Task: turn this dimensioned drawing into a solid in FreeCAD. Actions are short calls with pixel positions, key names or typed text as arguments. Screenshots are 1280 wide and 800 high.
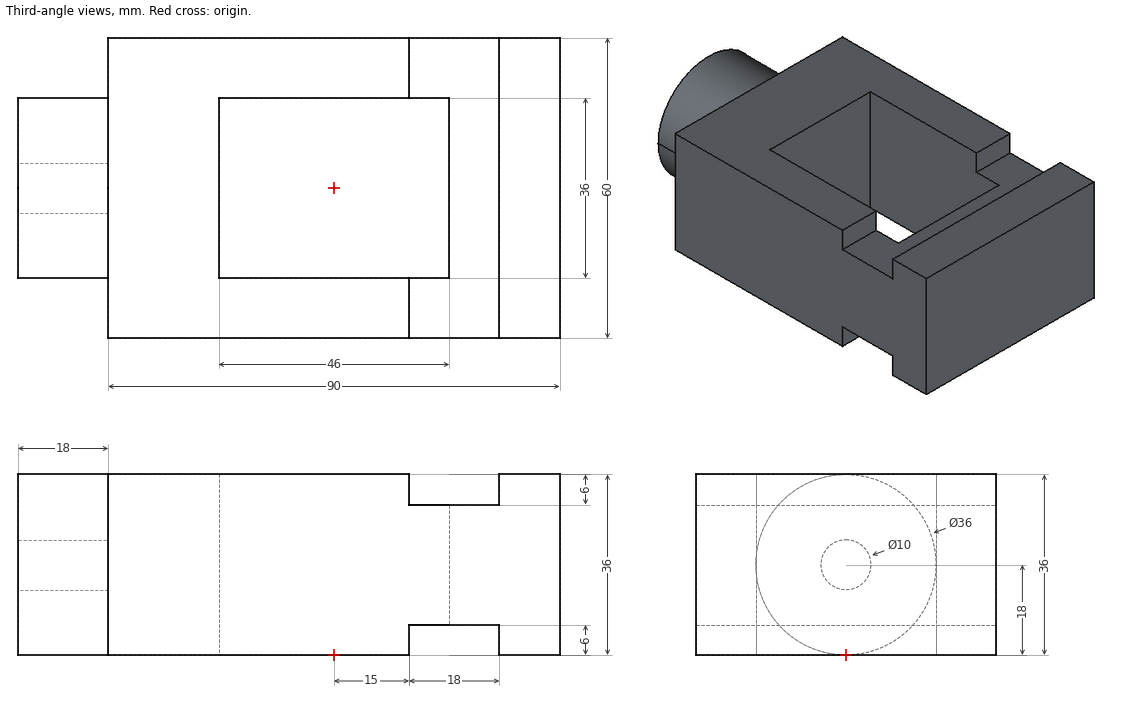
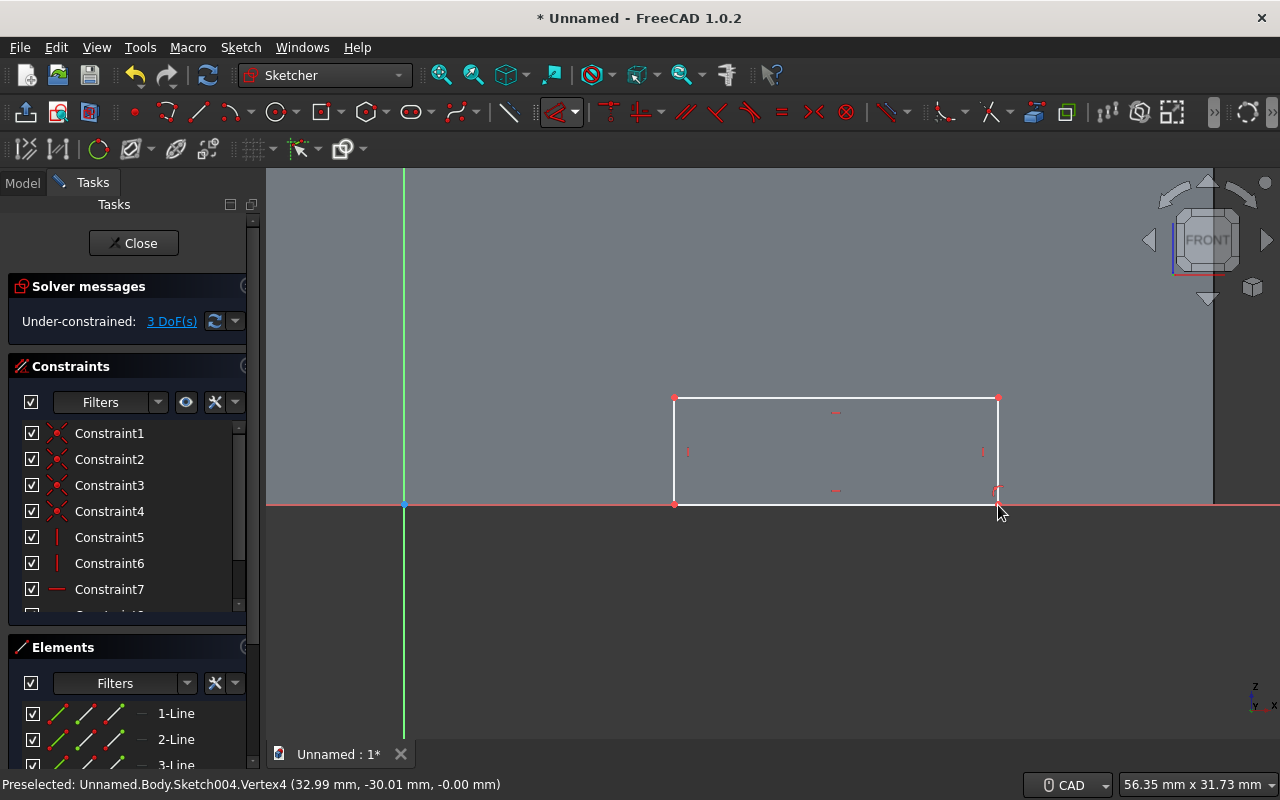
click(674, 430)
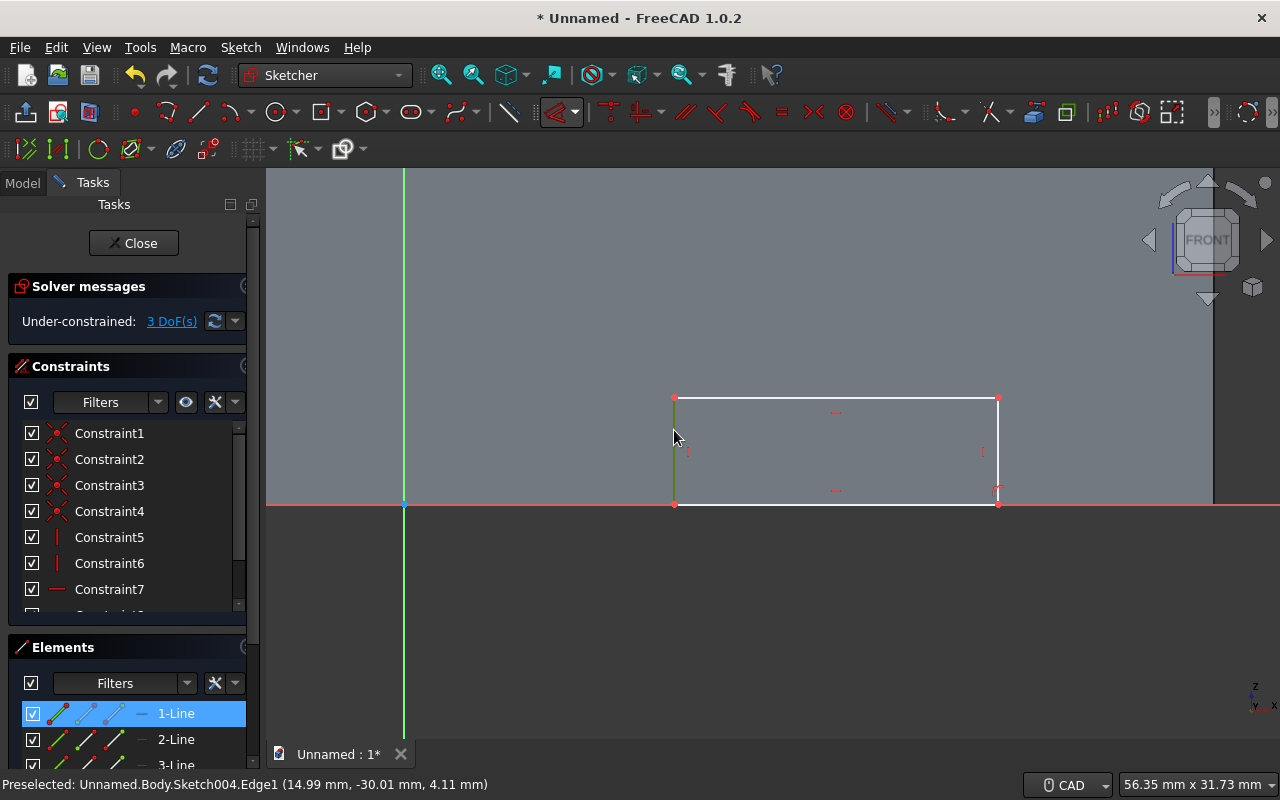
key(i)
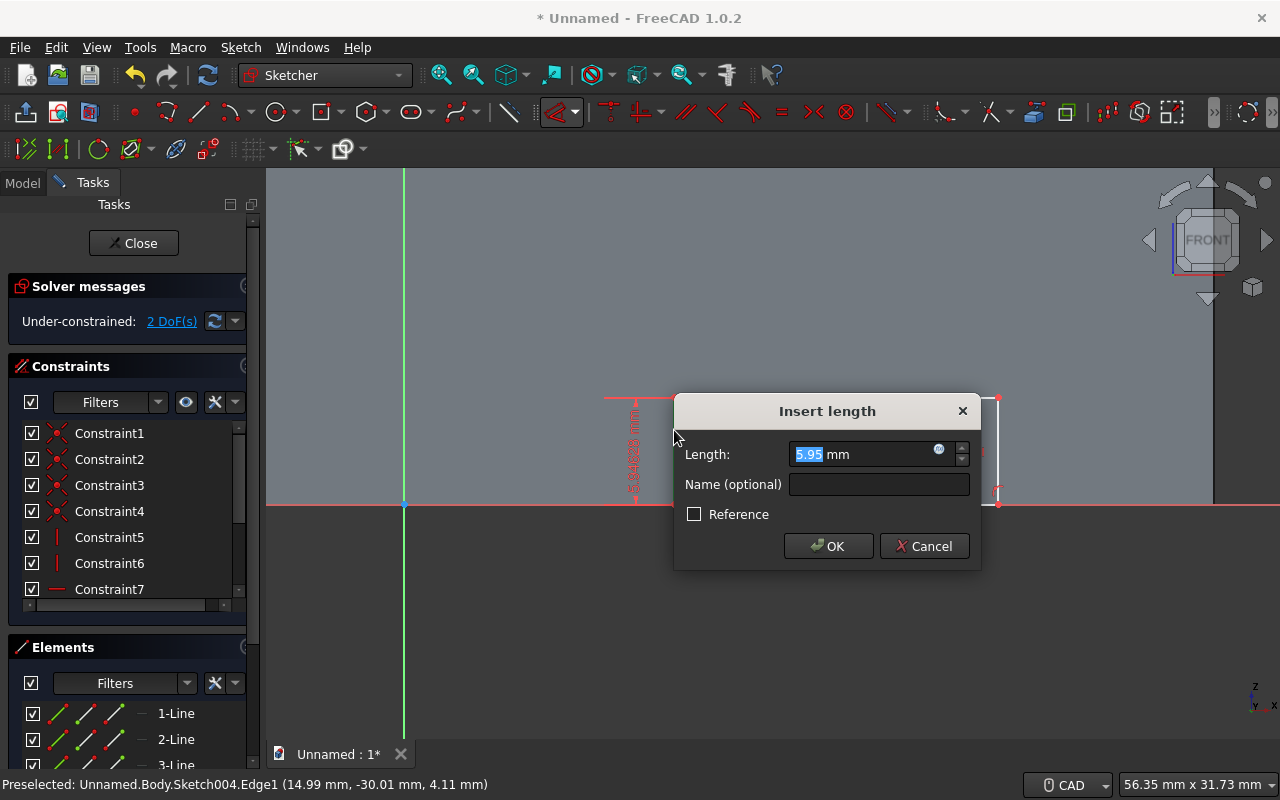
text(6)
key(Return)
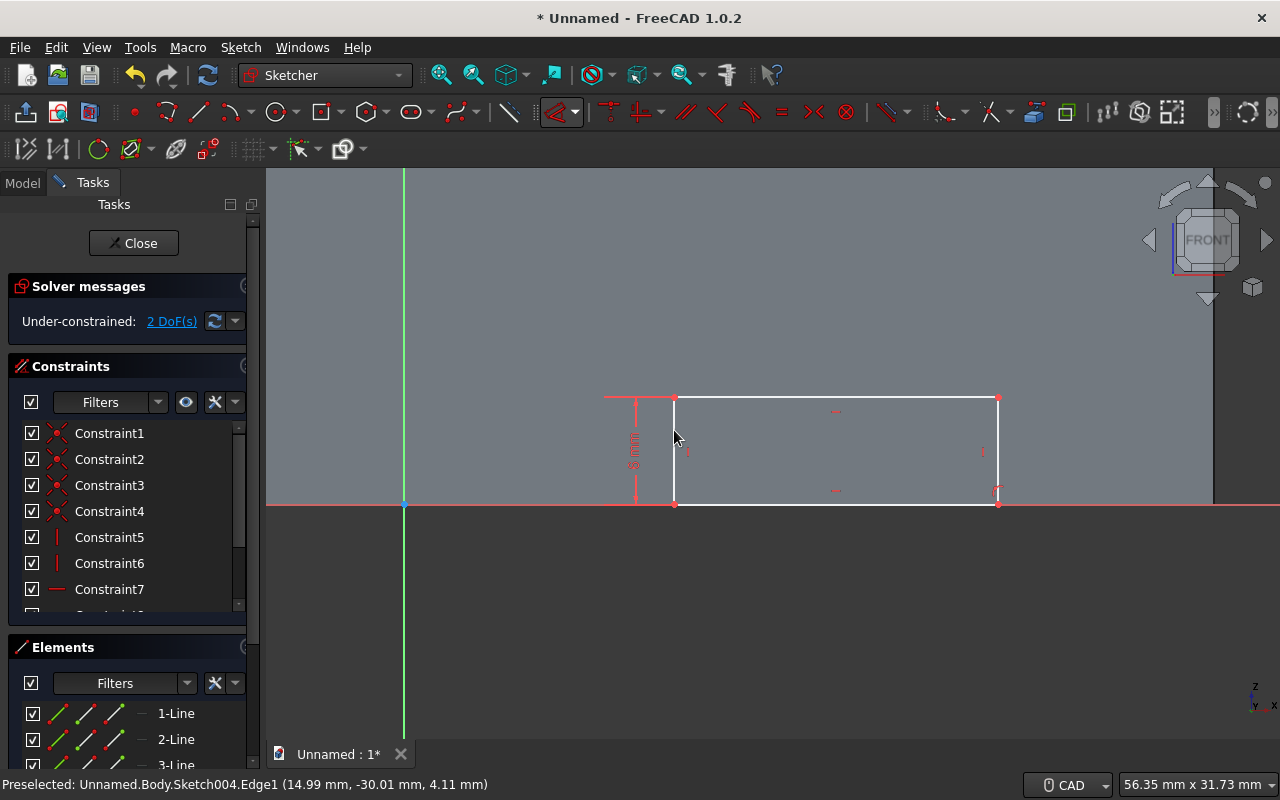
click(771, 505)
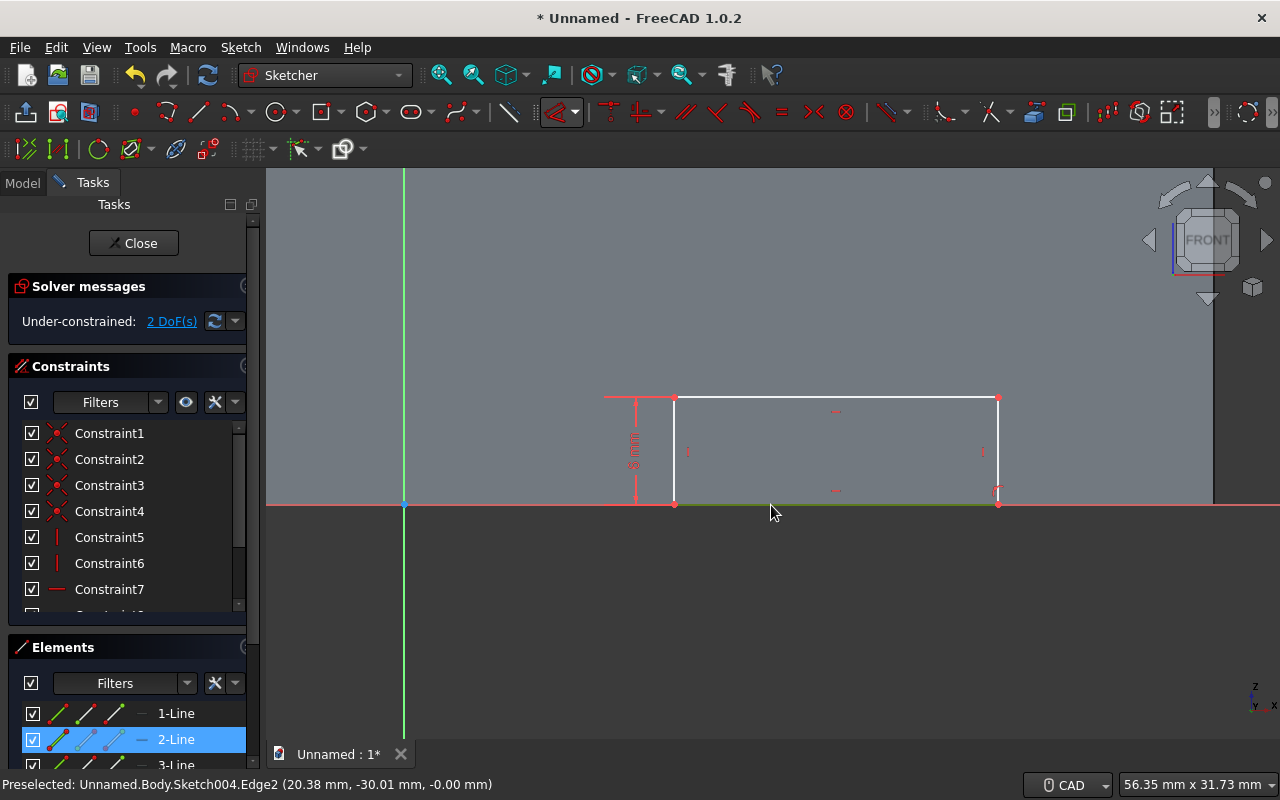
key(l)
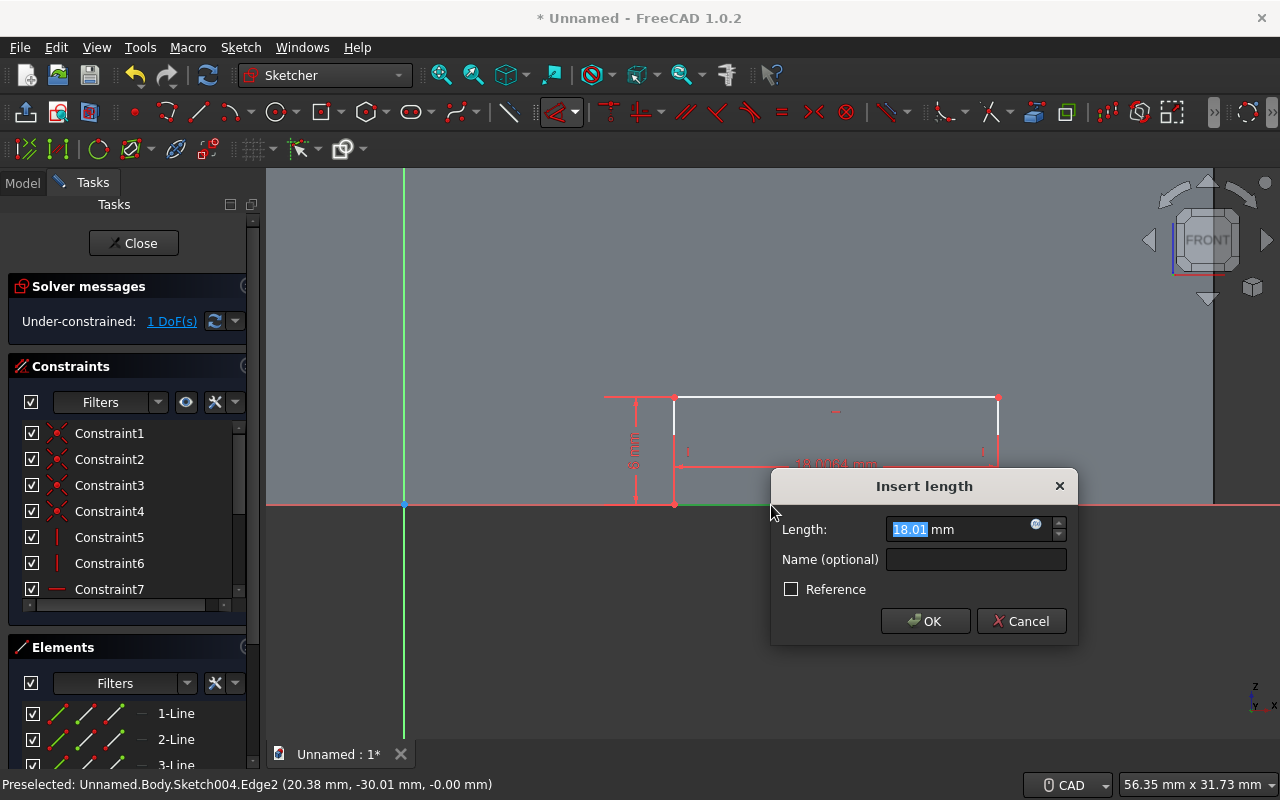
text(18)
key(Return)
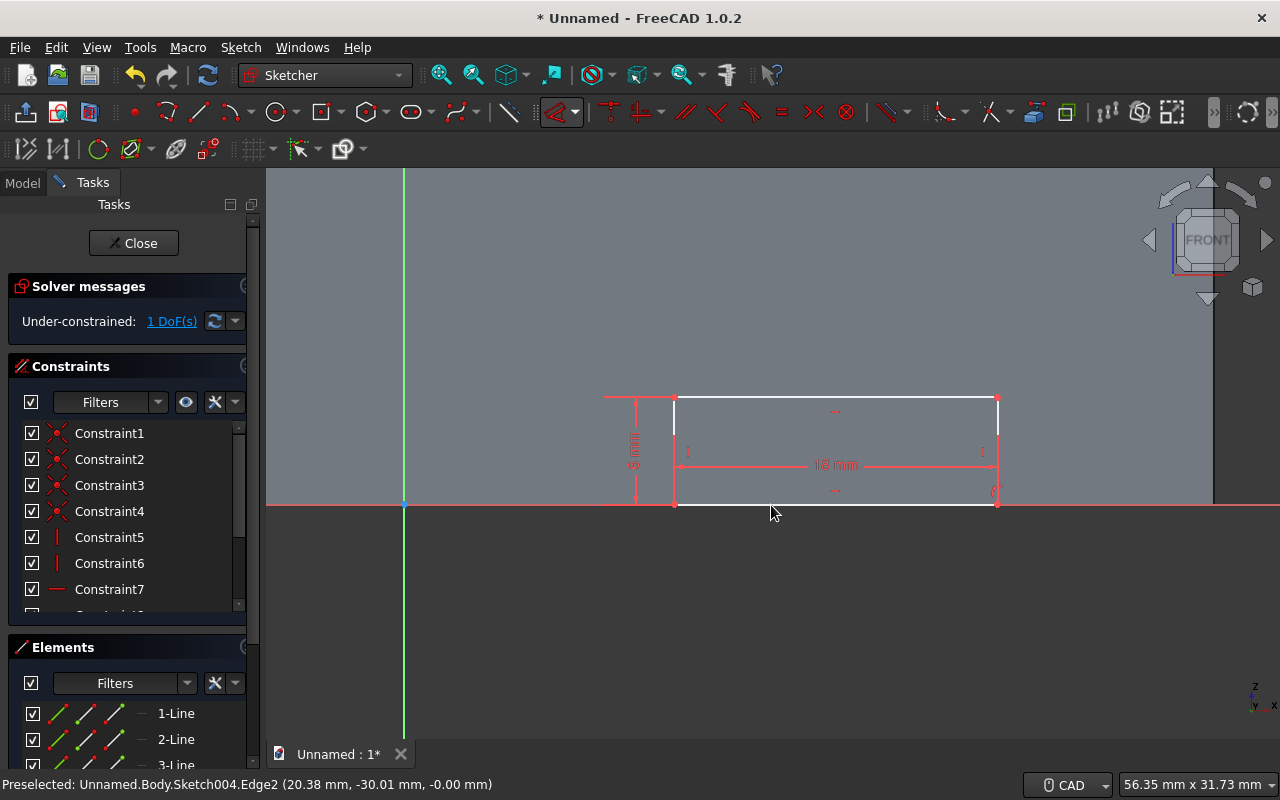
click(674, 397)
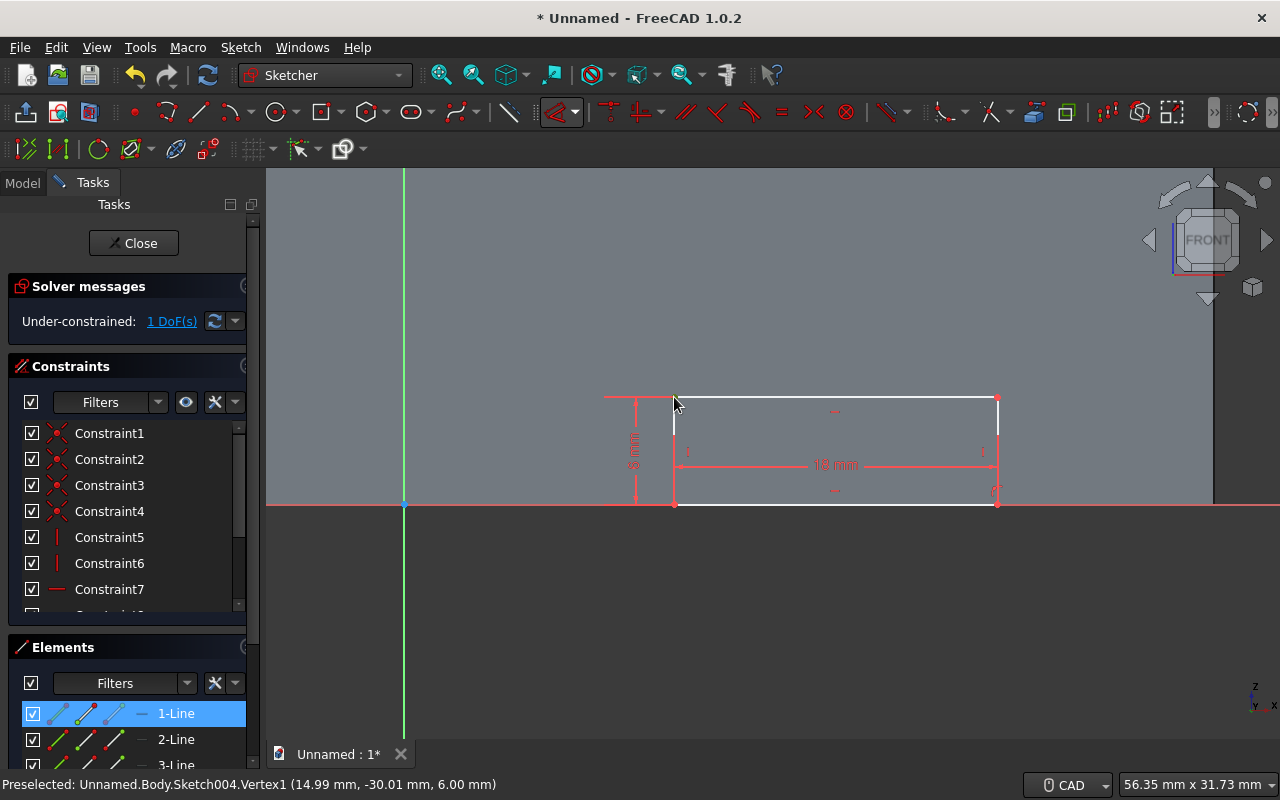
key(l)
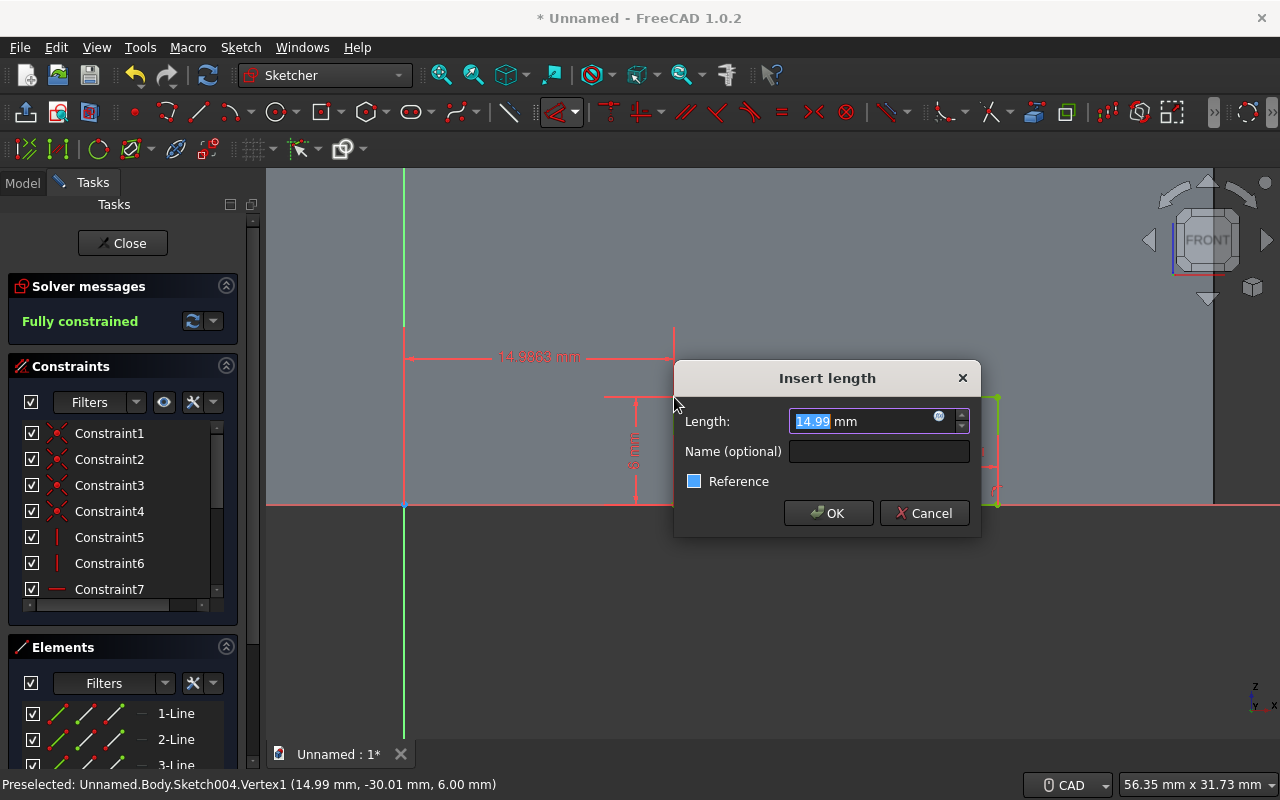
text(15)
key(Return)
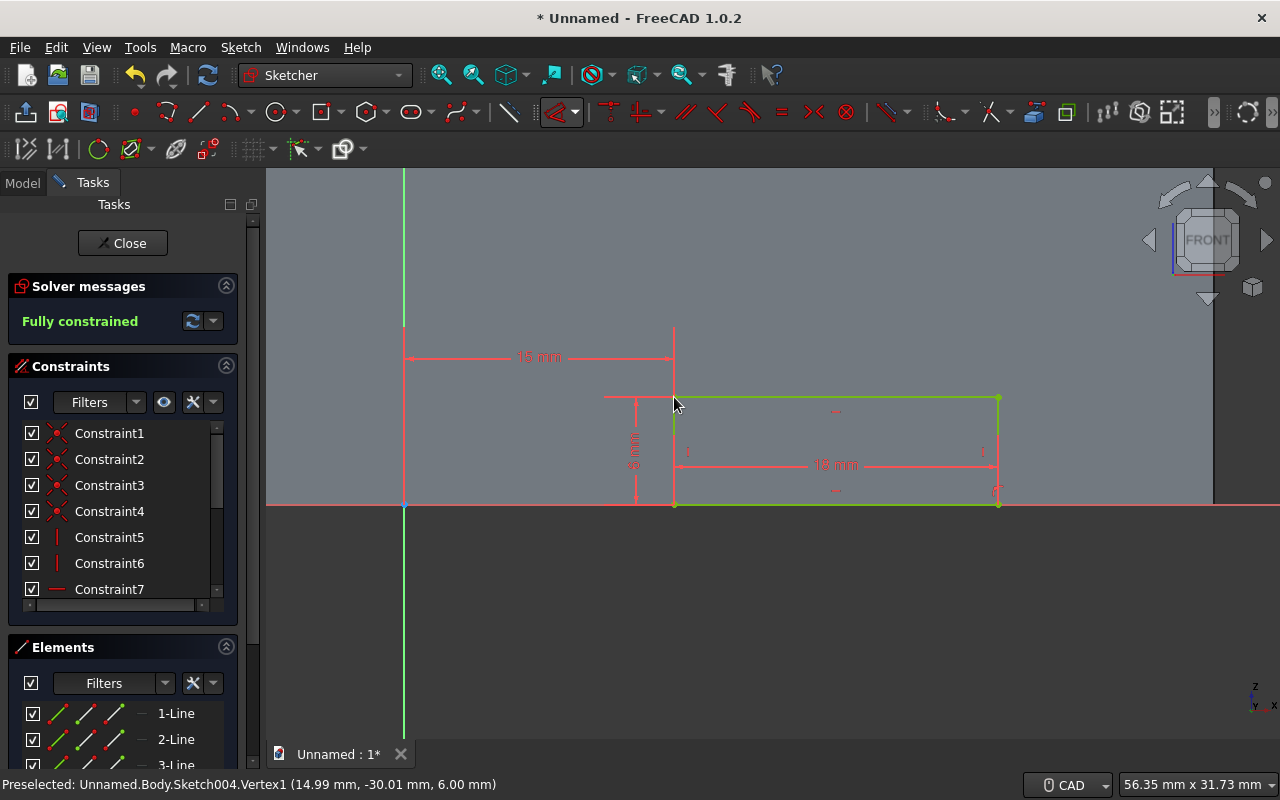
click(123, 243)